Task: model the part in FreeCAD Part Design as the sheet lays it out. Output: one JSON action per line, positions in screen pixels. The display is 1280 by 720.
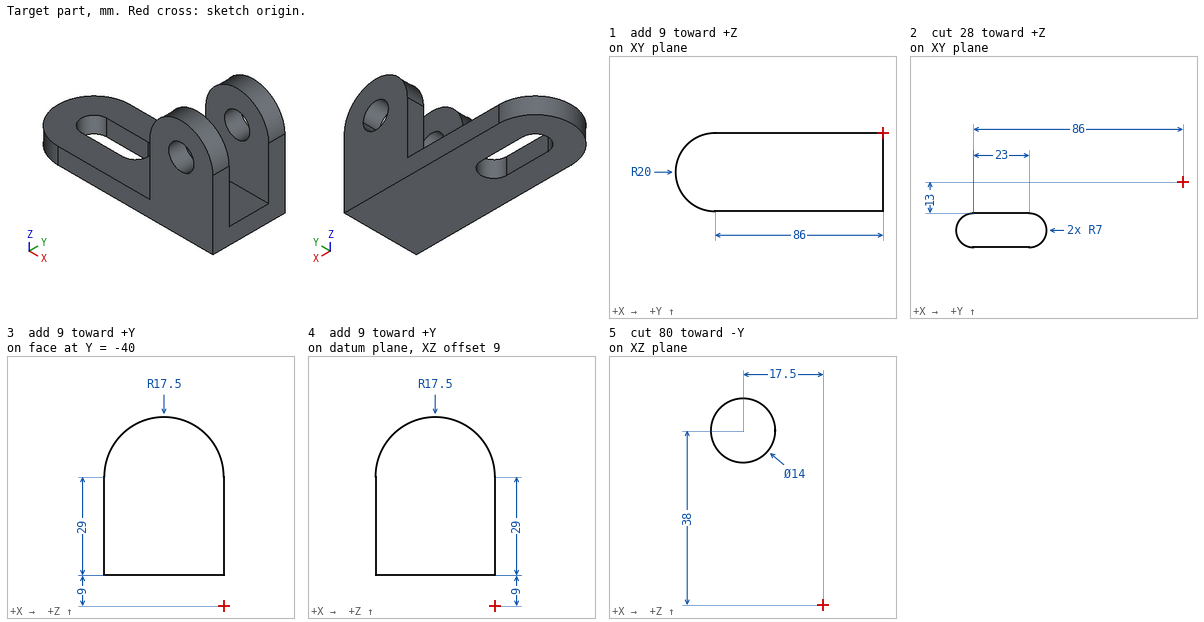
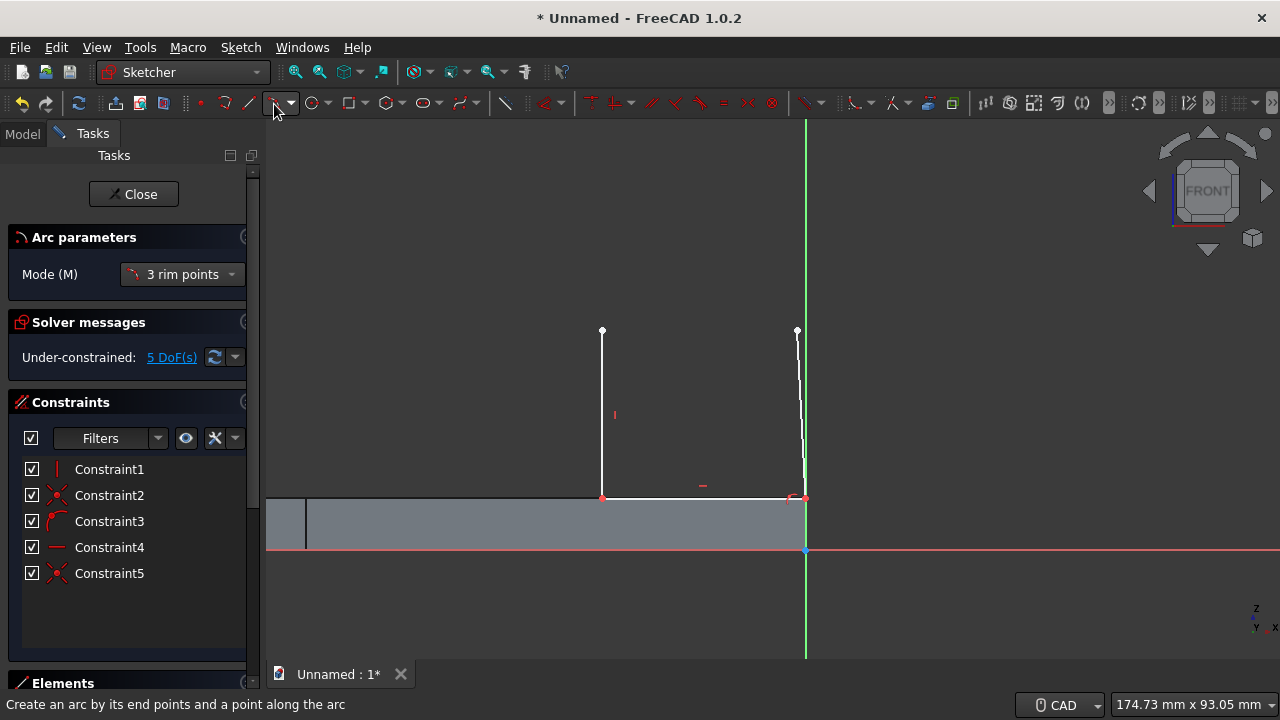
{"action": "left_click", "coordinate": [797, 331]}
{"action": "left_click", "coordinate": [602, 331]}
{"action": "left_click", "coordinate": [704, 228]}
{"action": "key", "text": "Escape"}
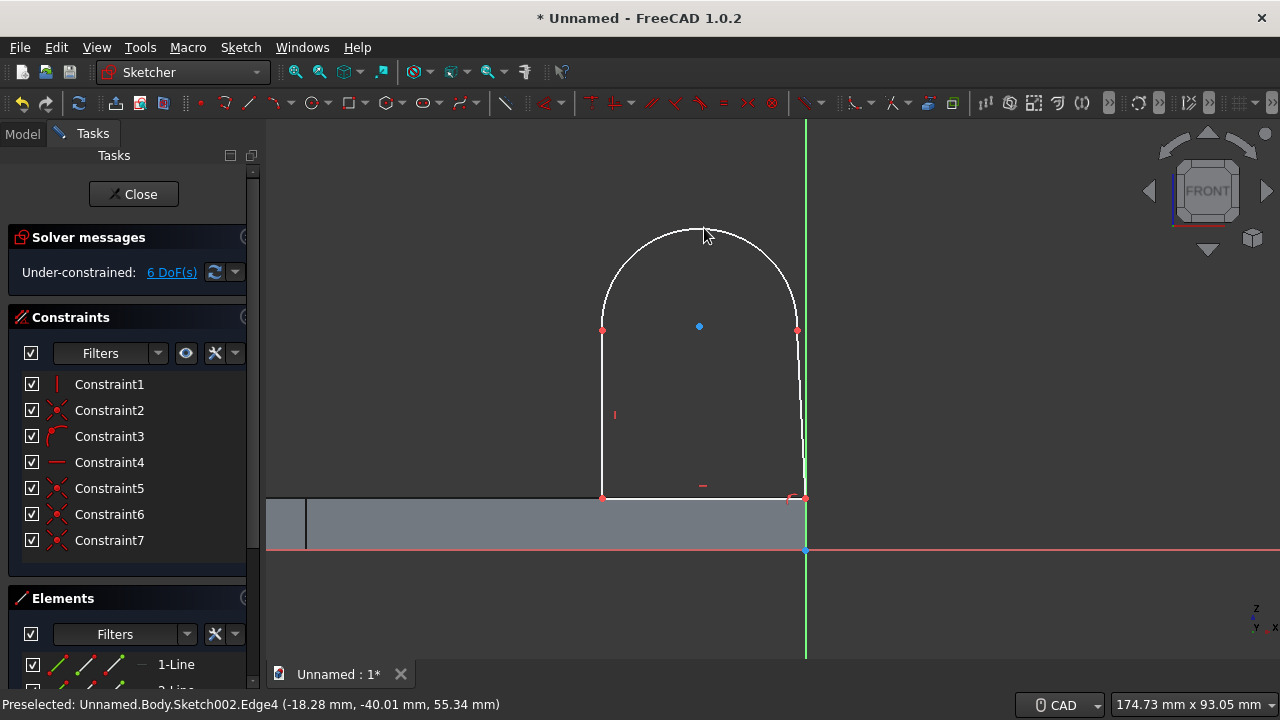
{"action": "left_click", "coordinate": [602, 381]}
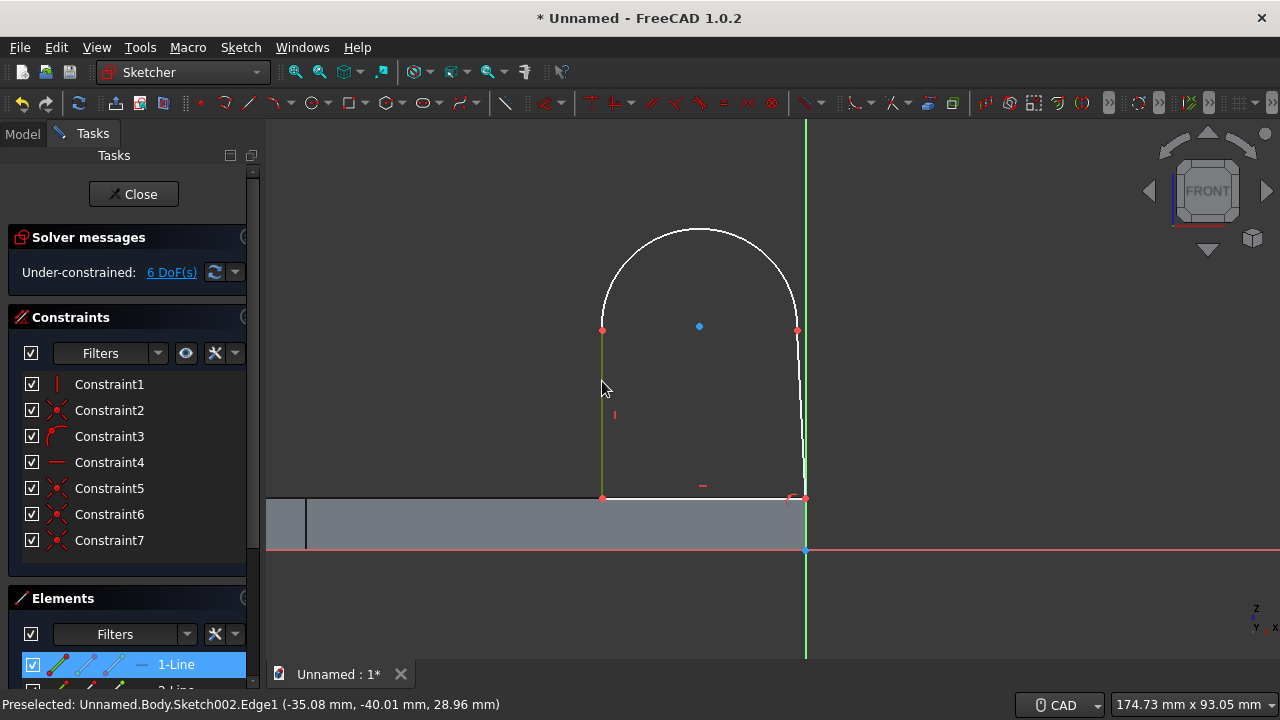
{"action": "left_click", "coordinate": [758, 249]}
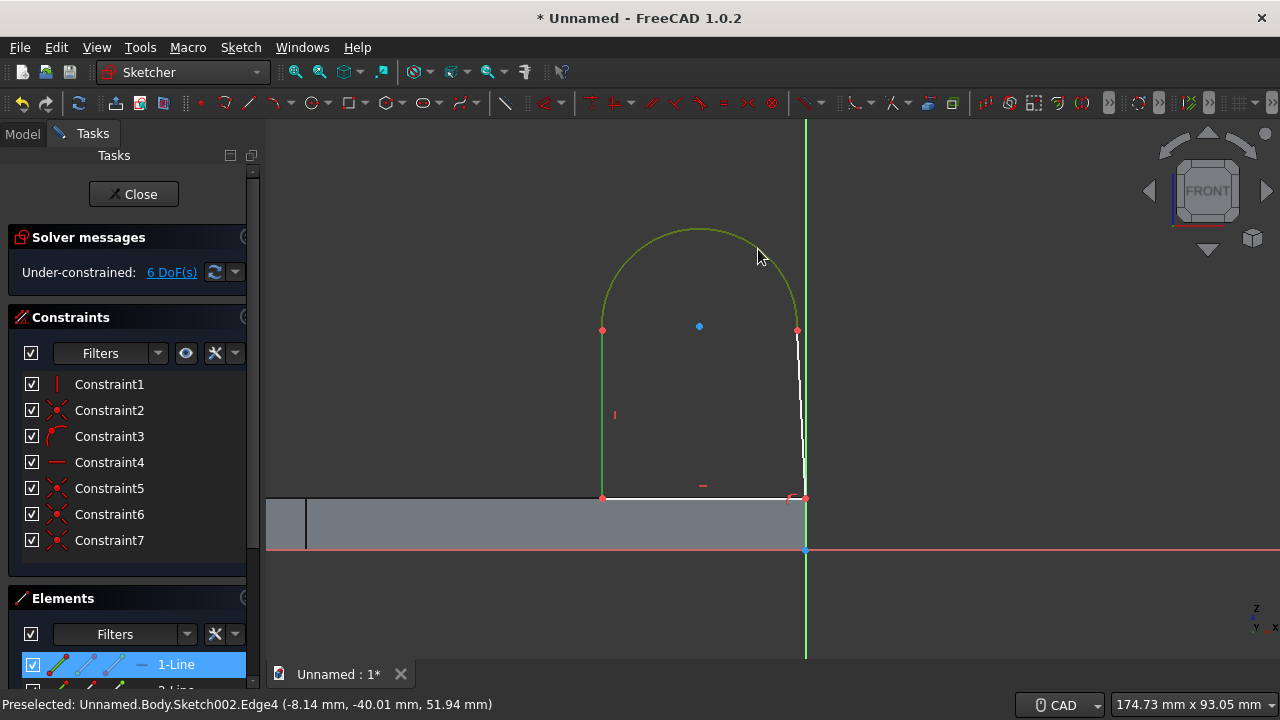
{"action": "left_click", "coordinate": [700, 104]}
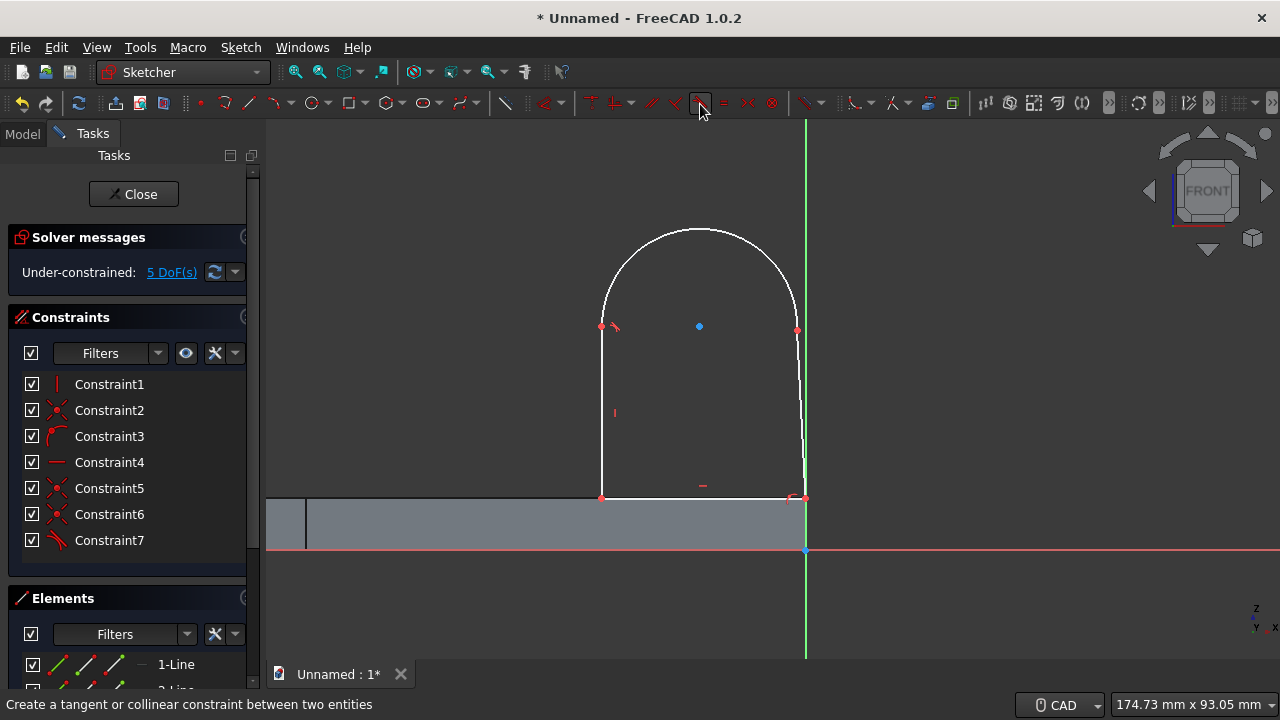
{"action": "left_click", "coordinate": [803, 449]}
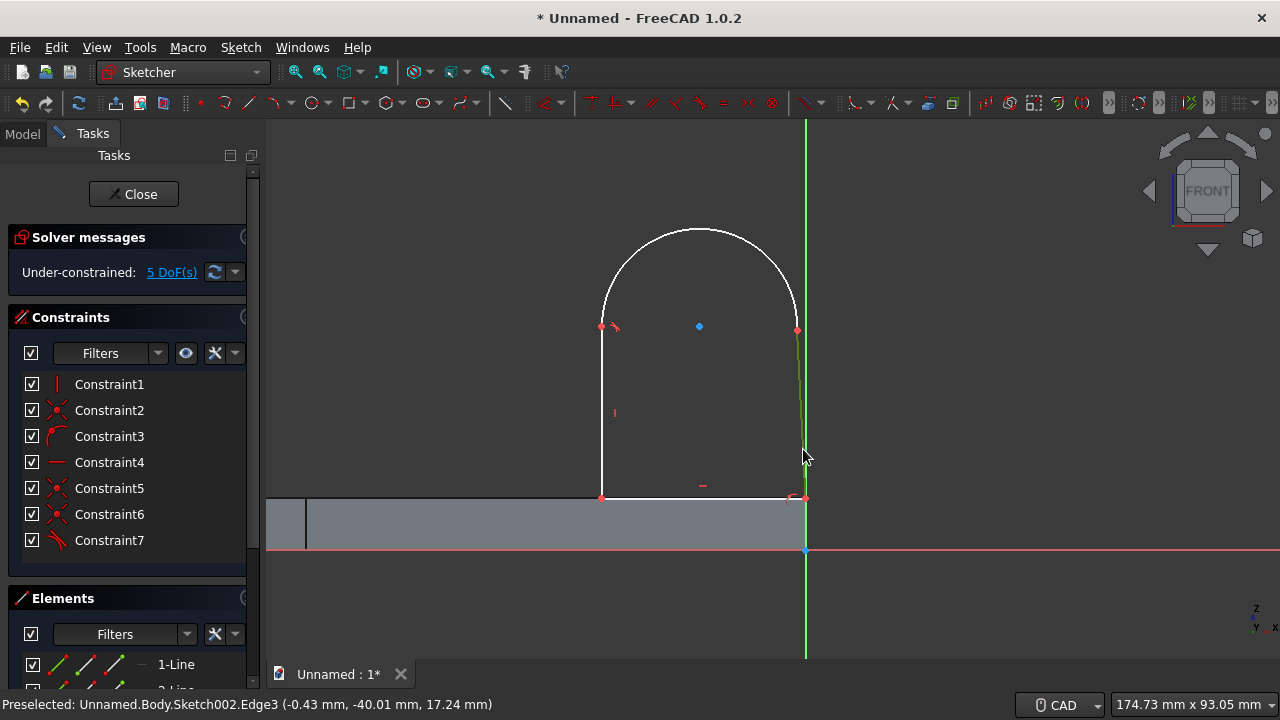
{"action": "left_click", "coordinate": [759, 249]}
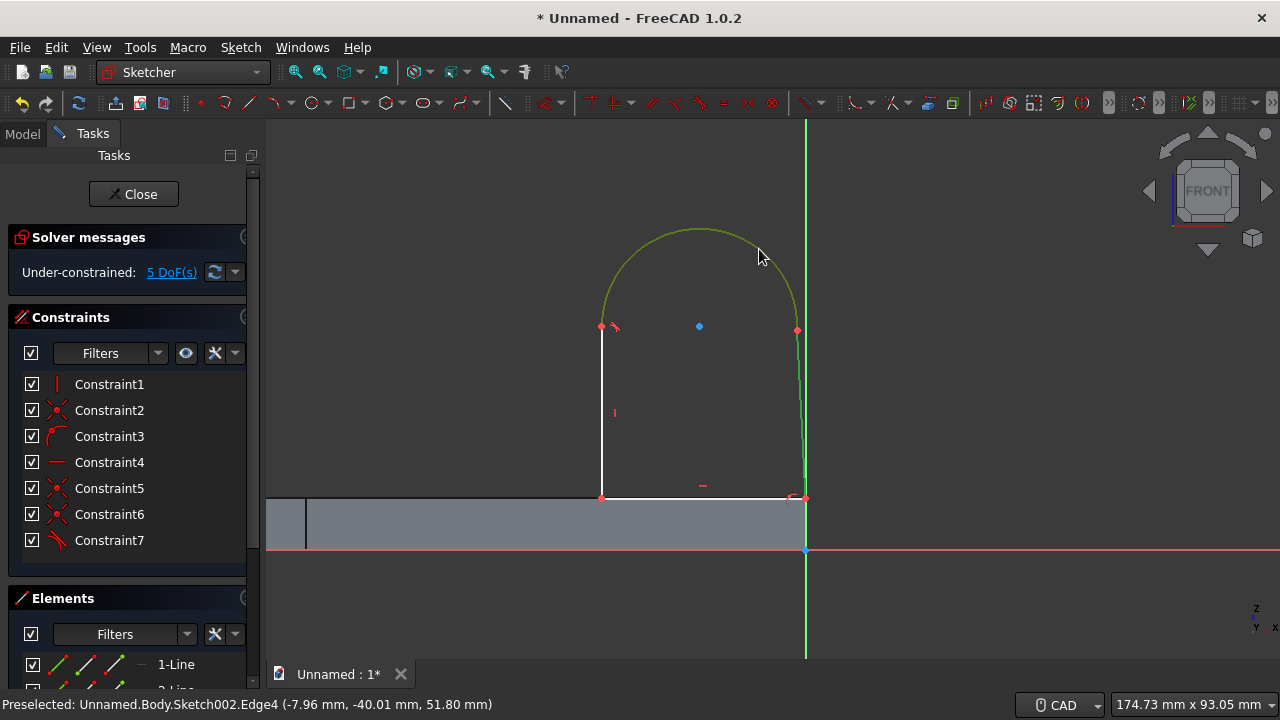
{"action": "left_click", "coordinate": [700, 104]}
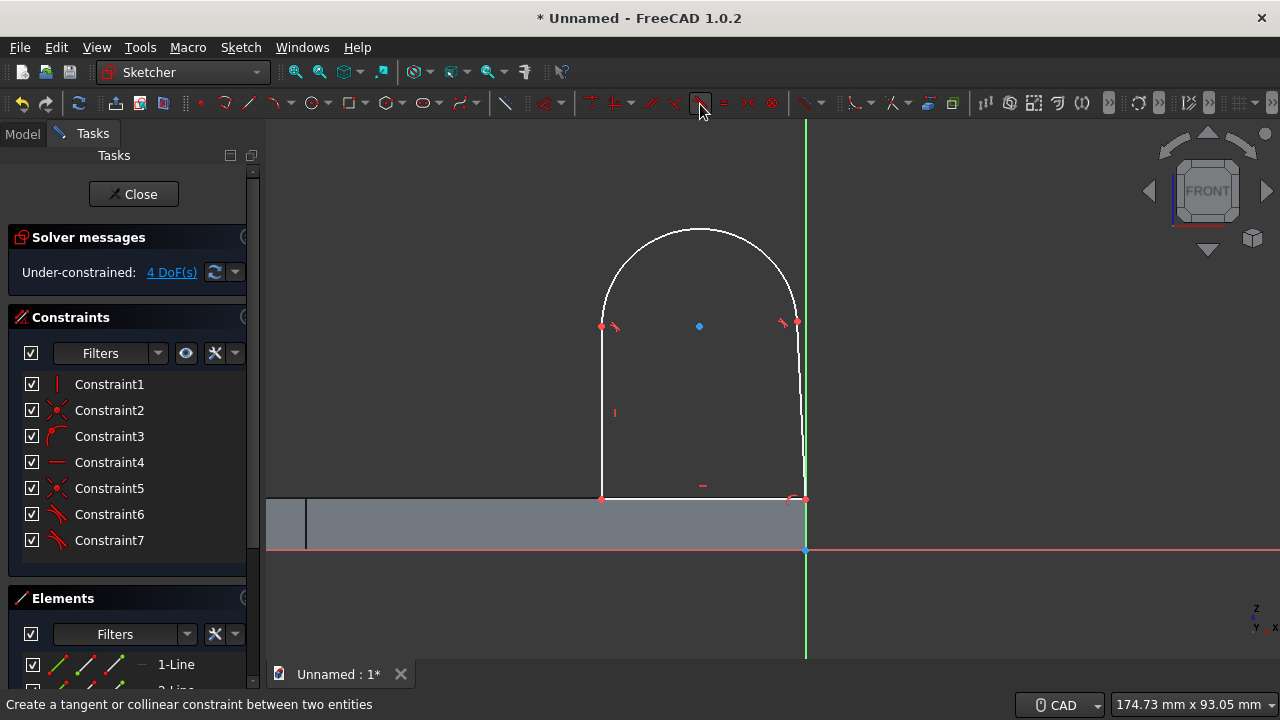
{"action": "left_click", "coordinate": [803, 446]}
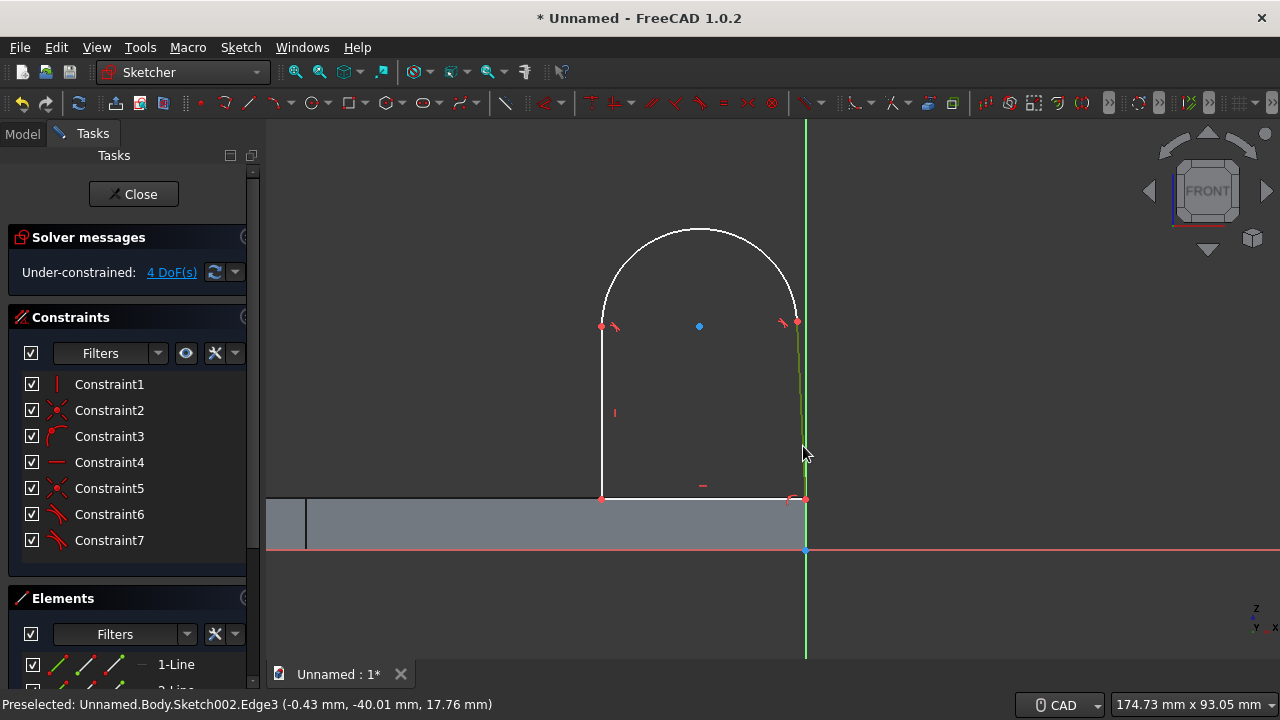
{"action": "left_click", "coordinate": [634, 104]}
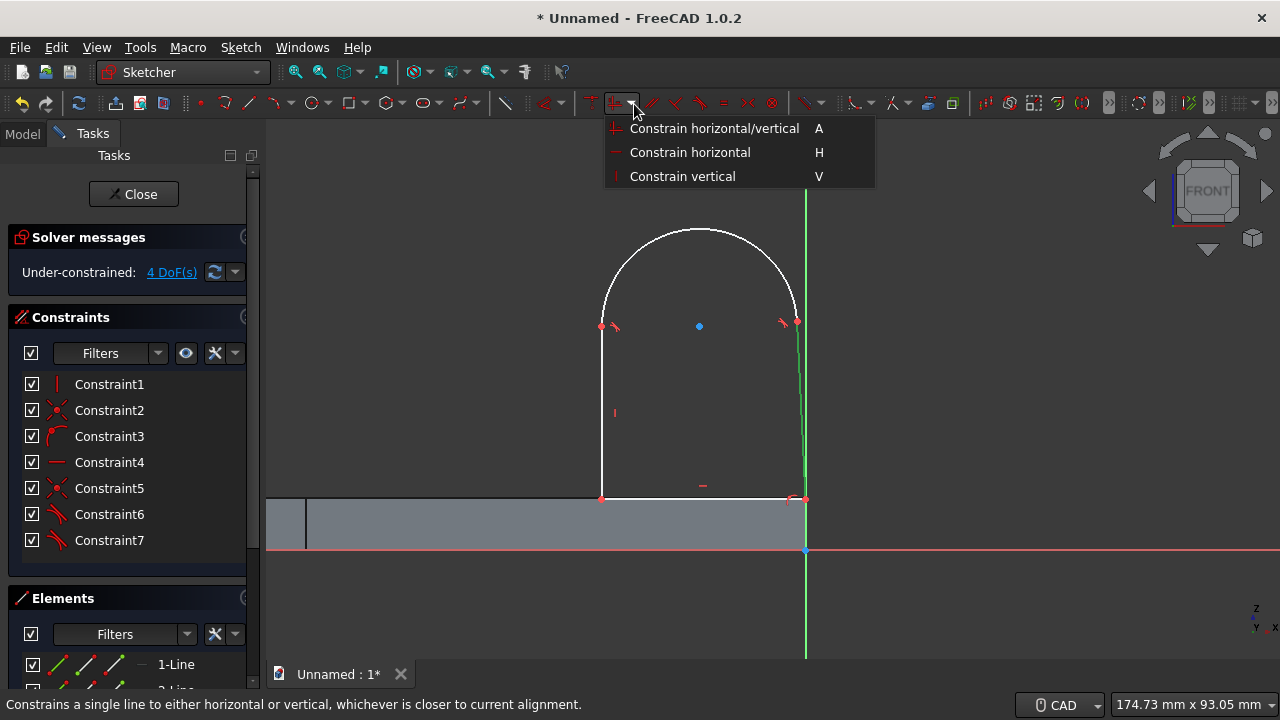
{"action": "left_click", "coordinate": [740, 176]}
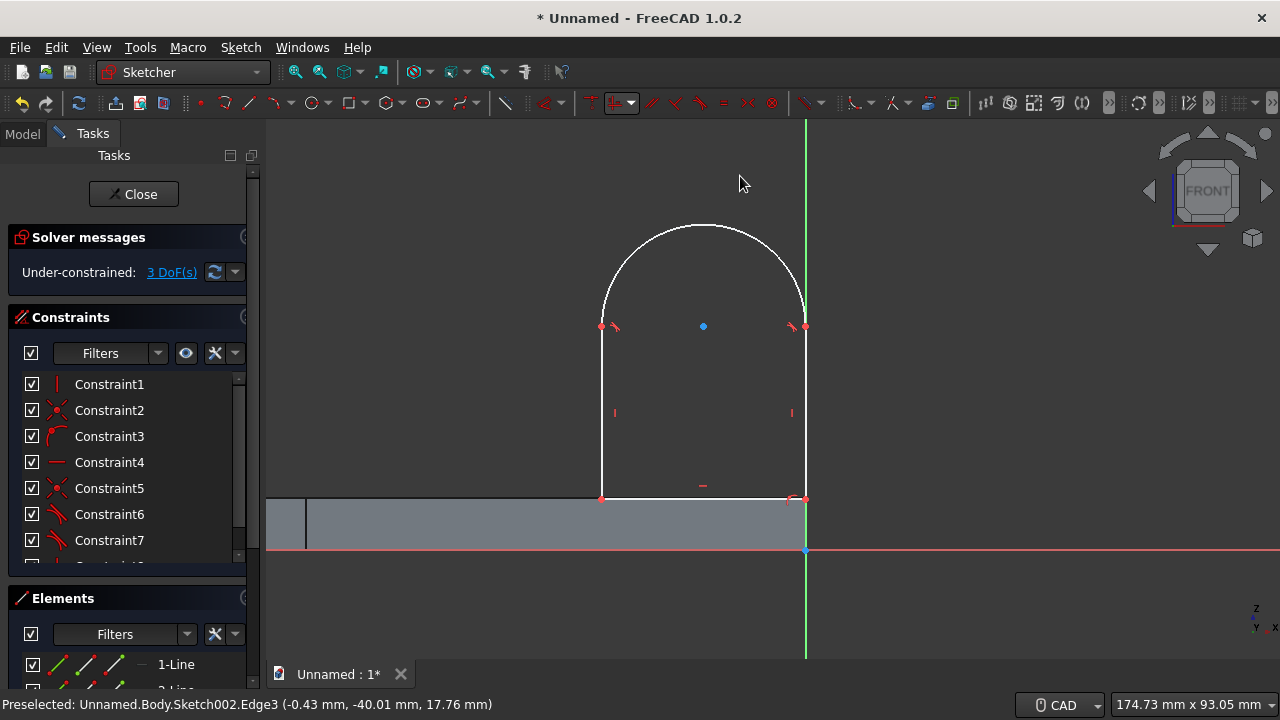
{"action": "left_click", "coordinate": [544, 104]}